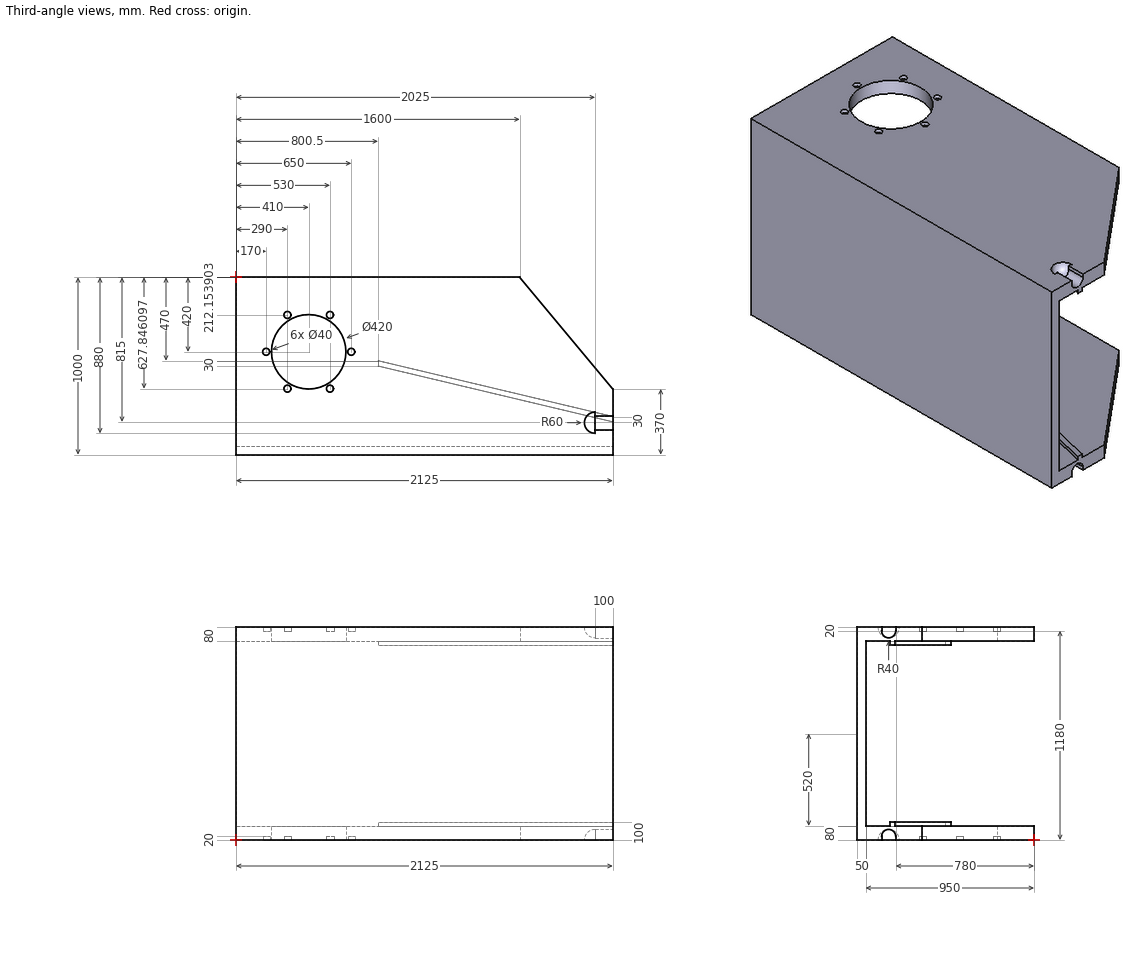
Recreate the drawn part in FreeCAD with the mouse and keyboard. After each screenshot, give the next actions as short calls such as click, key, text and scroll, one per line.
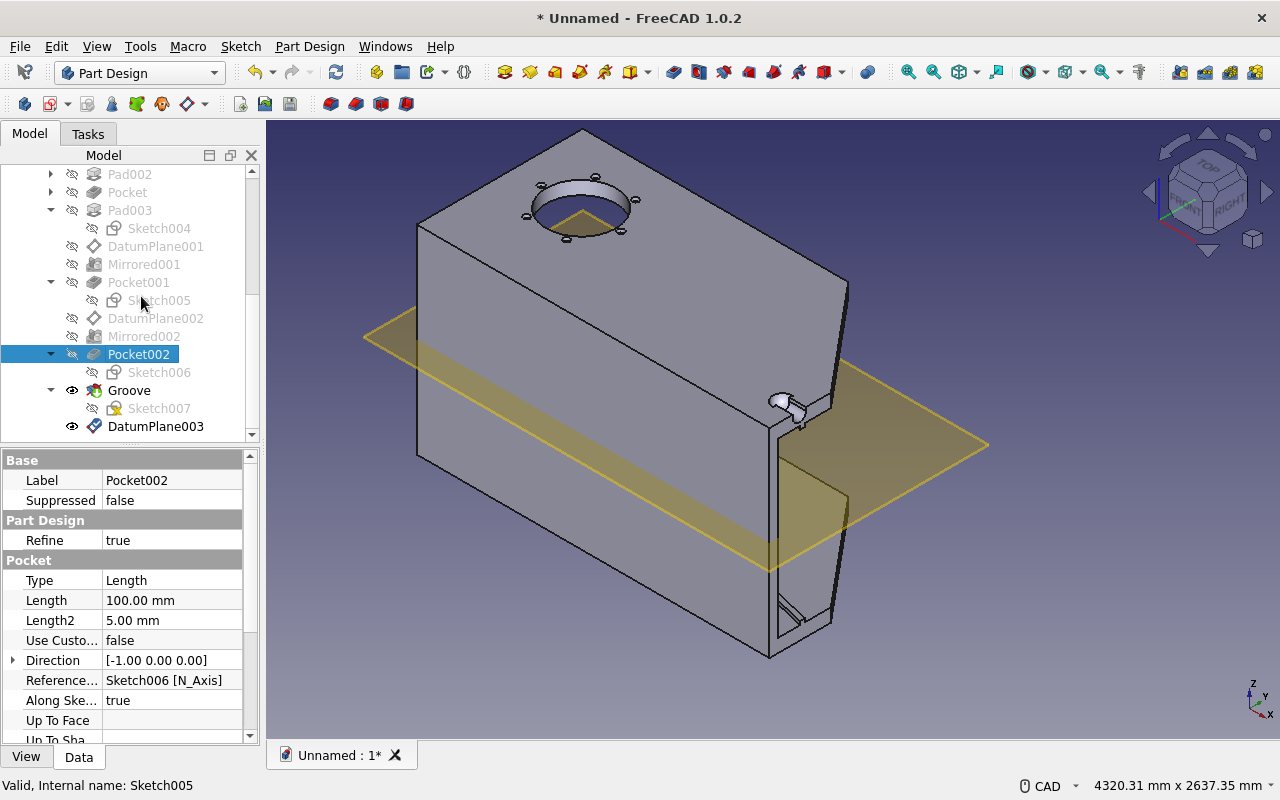
click(117, 390, ctrl)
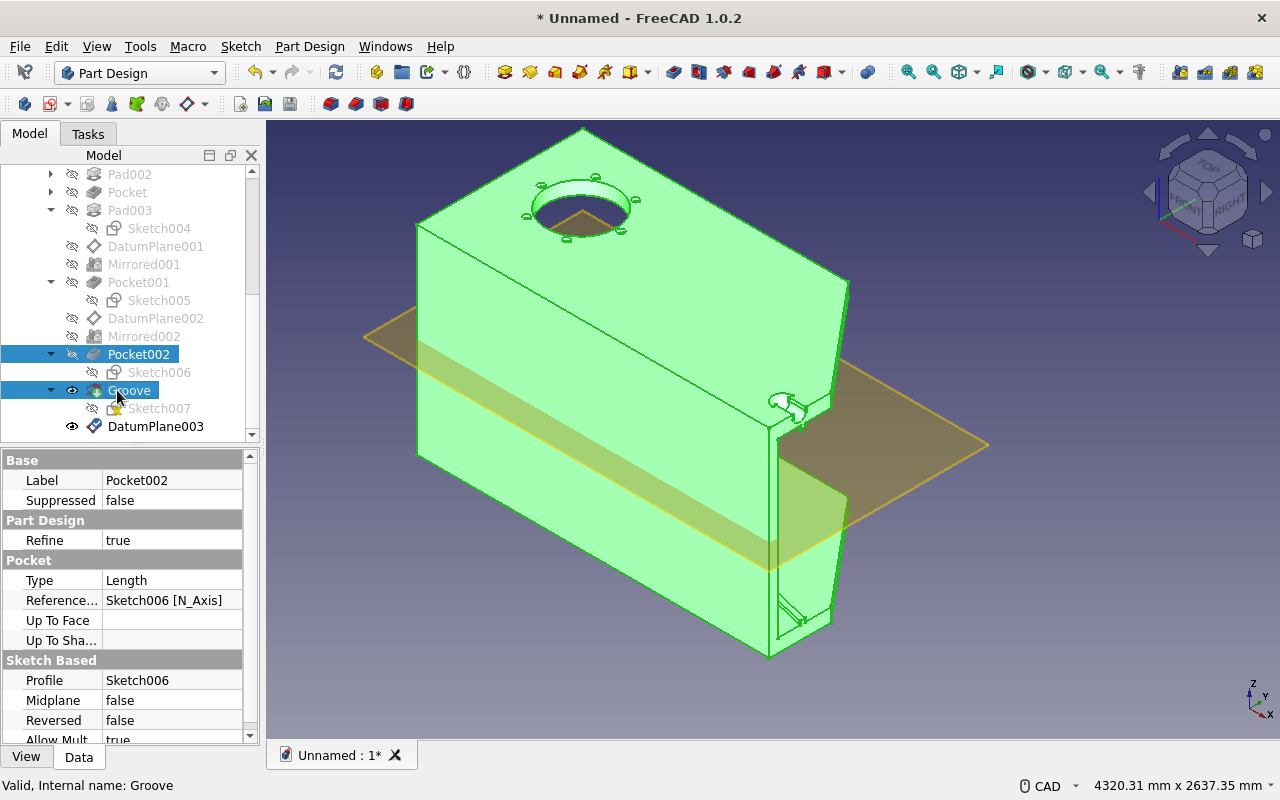
click(1180, 72)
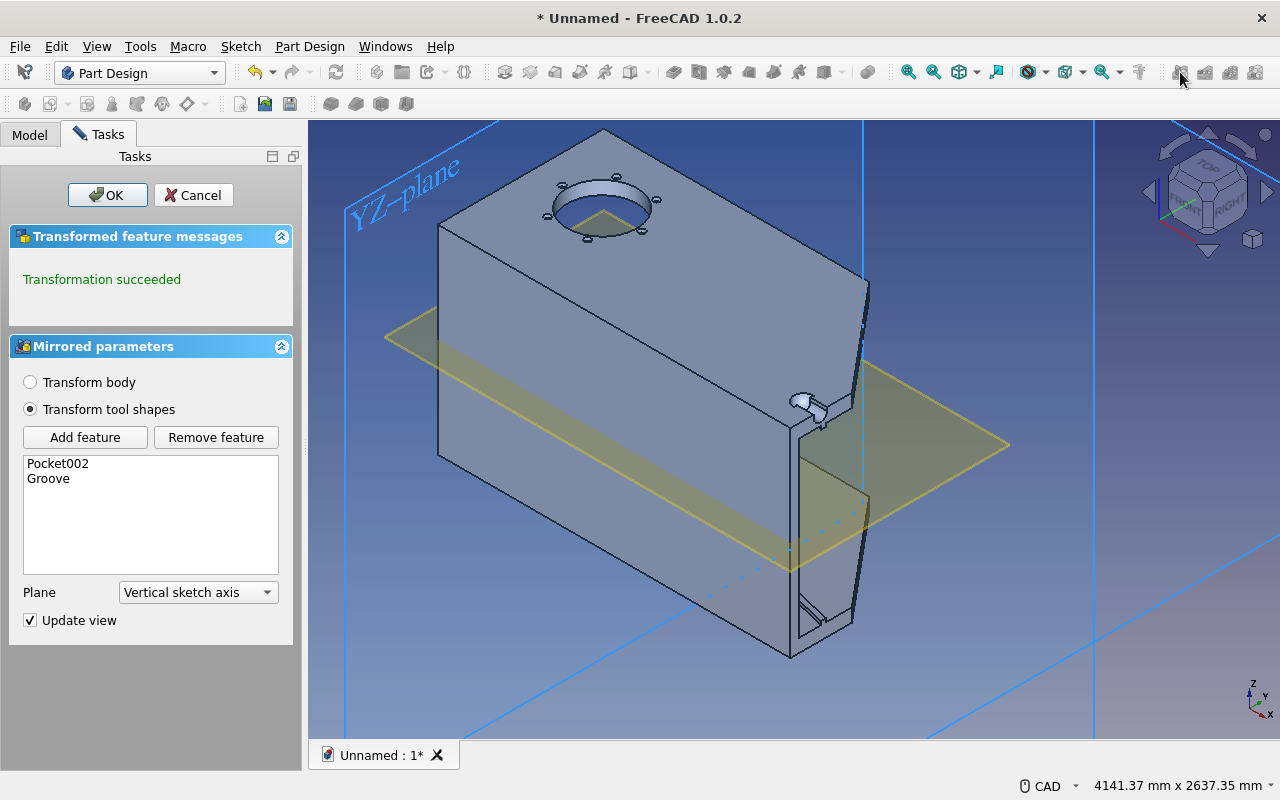
click(199, 592)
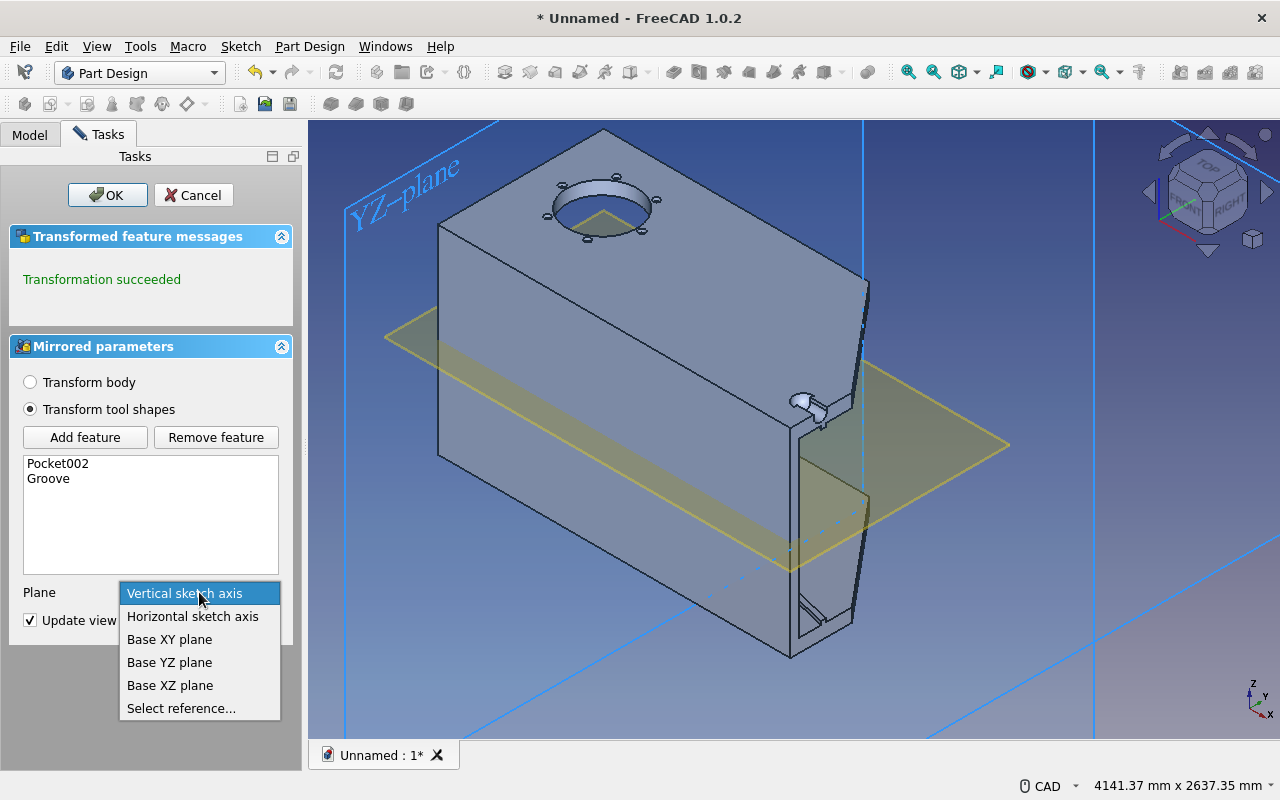
click(198, 708)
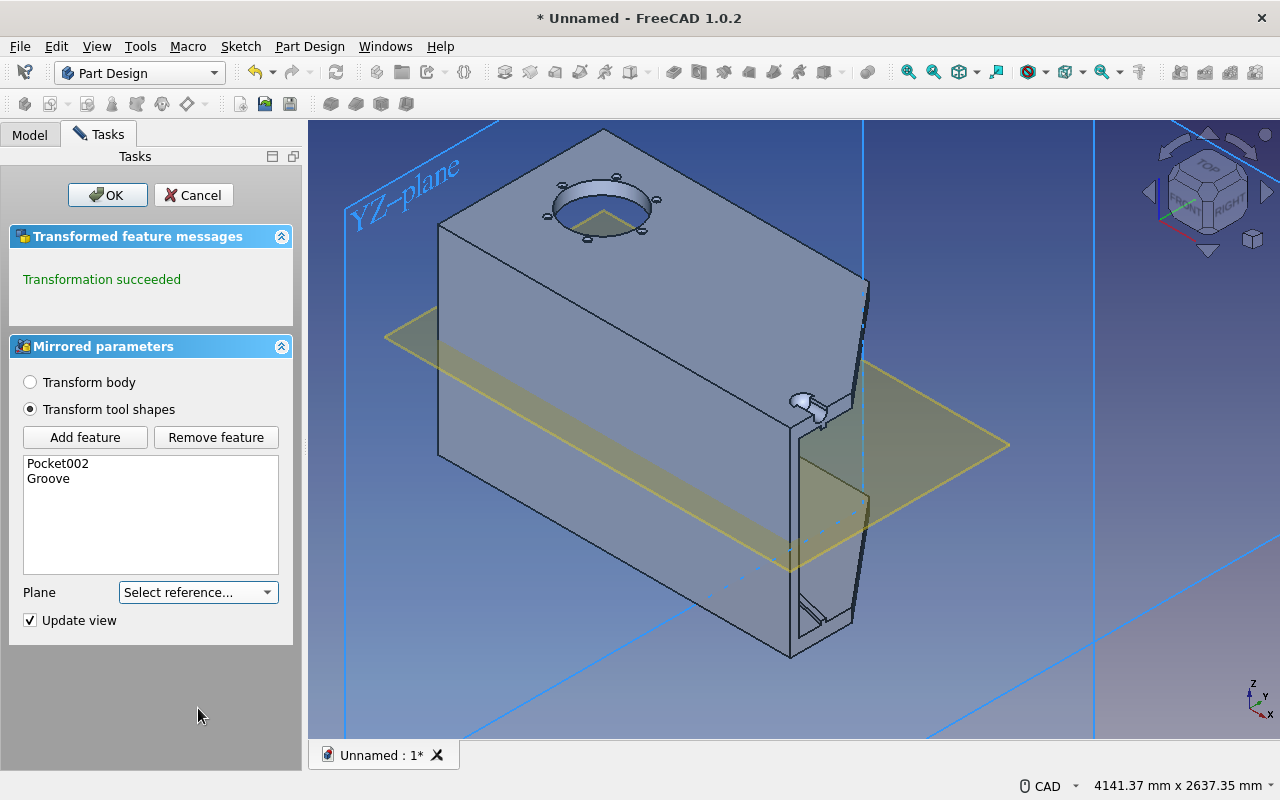
click(30, 134)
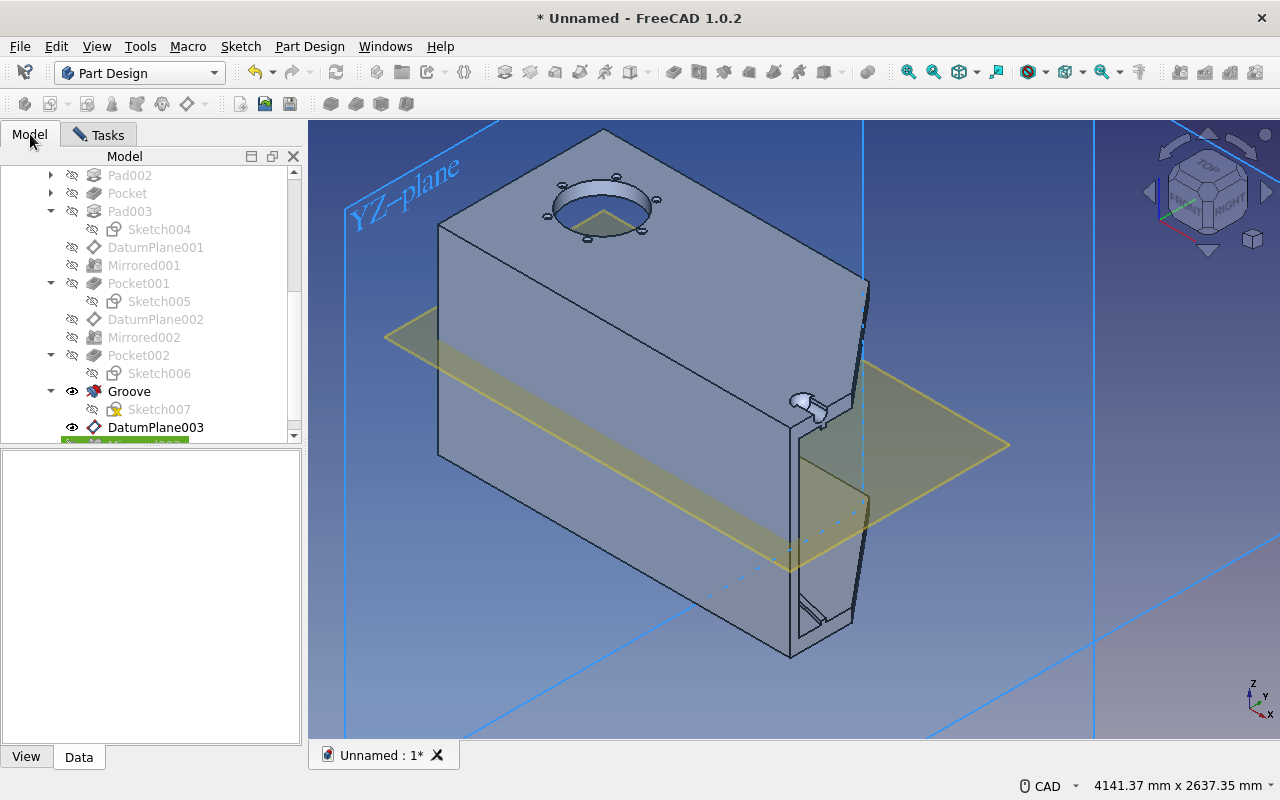
click(117, 427)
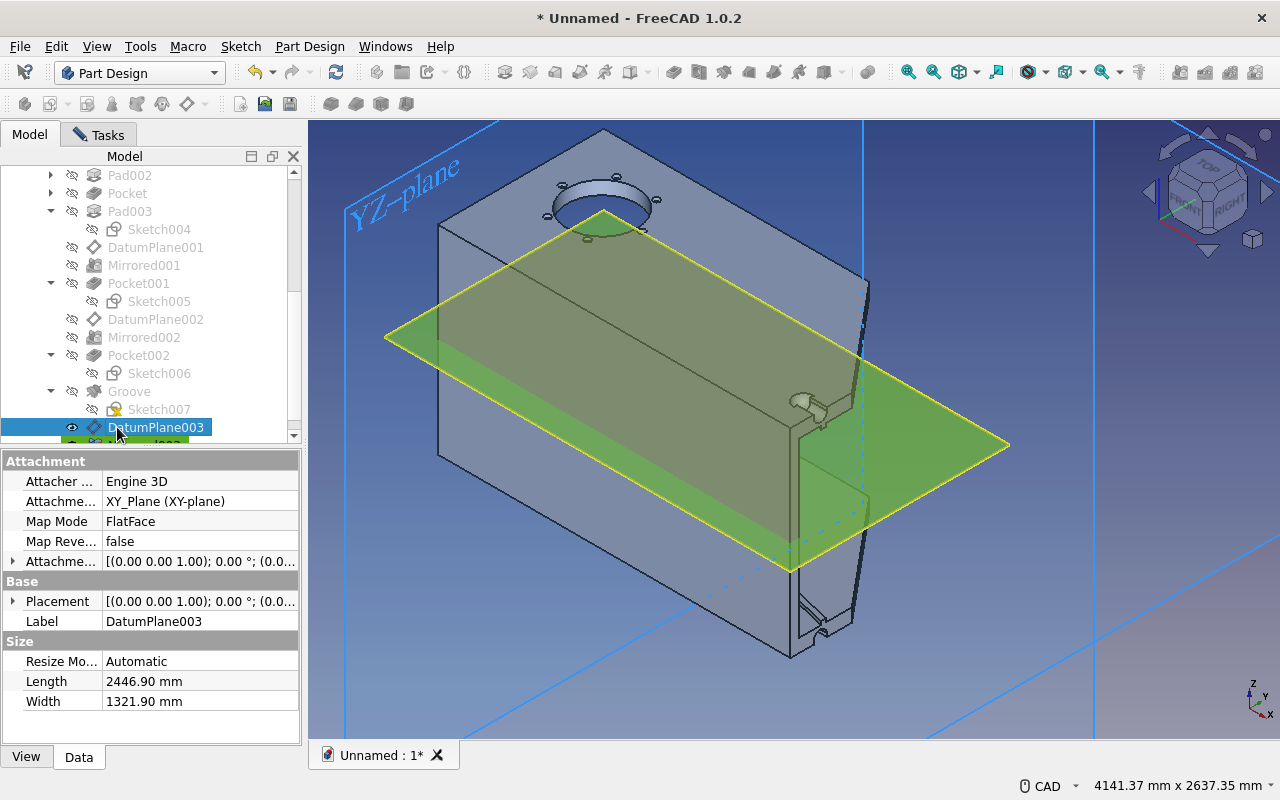
click(98, 134)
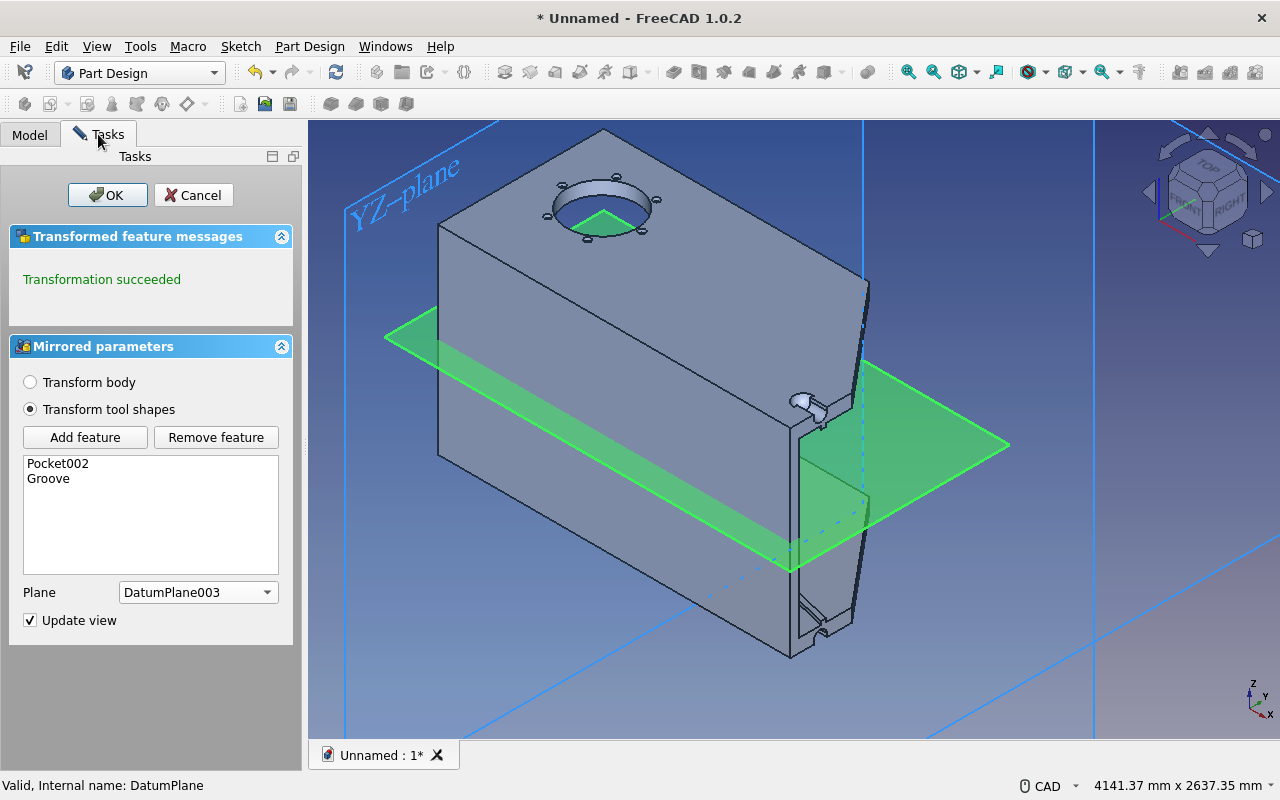
click(108, 195)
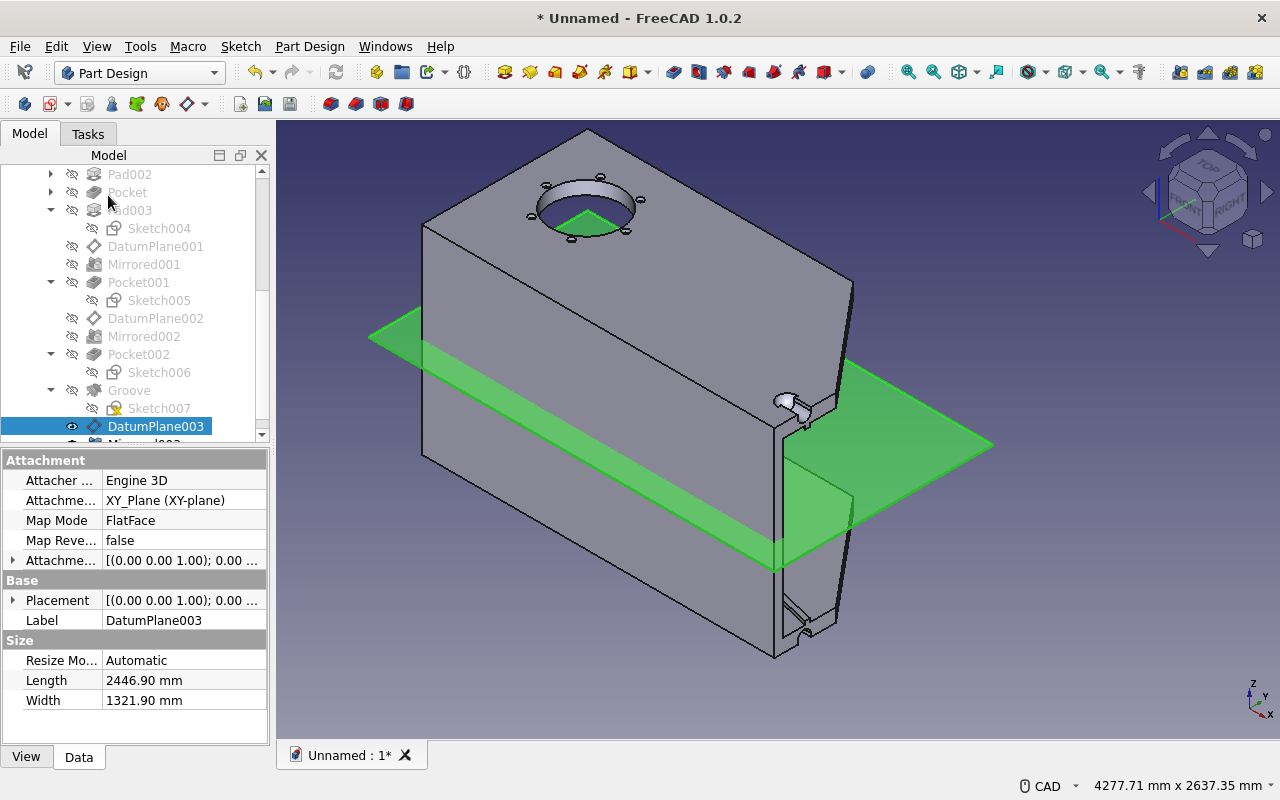
click(117, 426)
key(space)